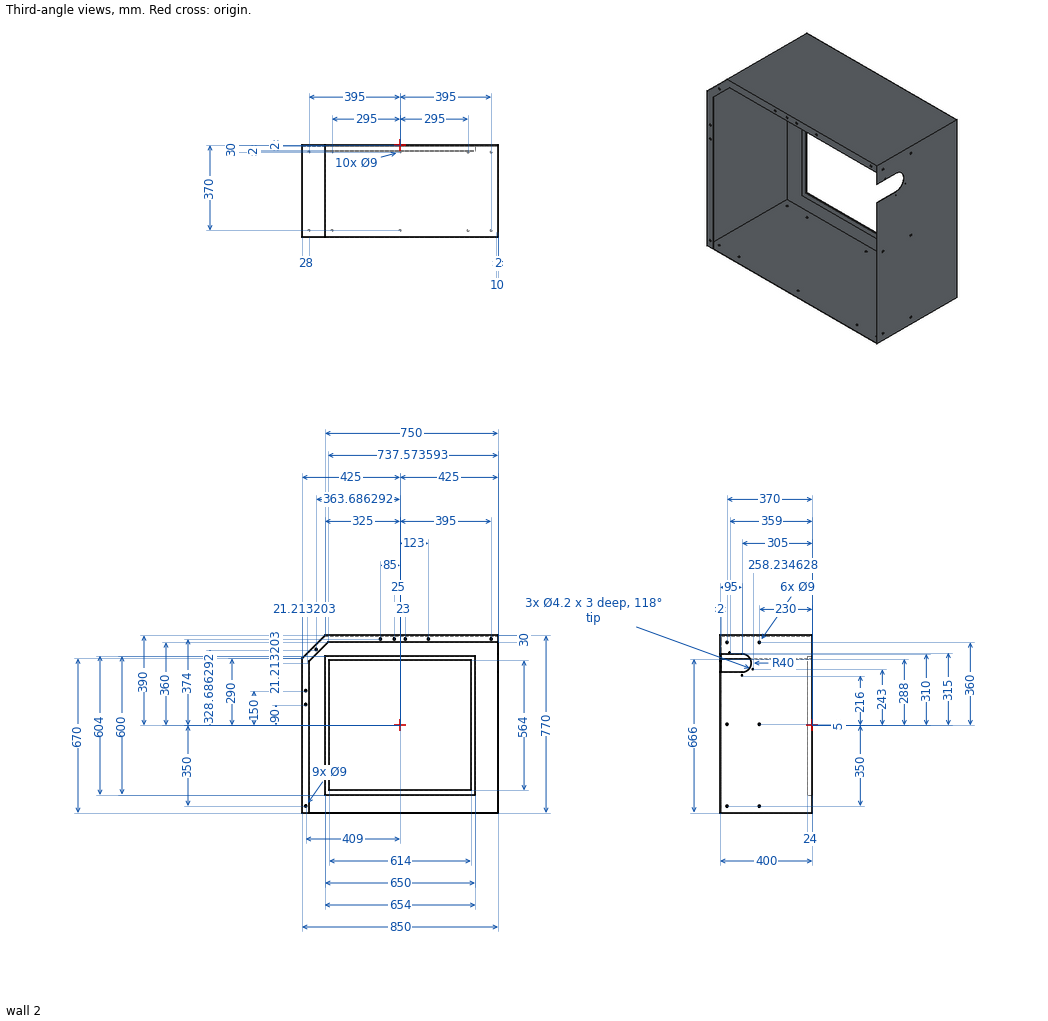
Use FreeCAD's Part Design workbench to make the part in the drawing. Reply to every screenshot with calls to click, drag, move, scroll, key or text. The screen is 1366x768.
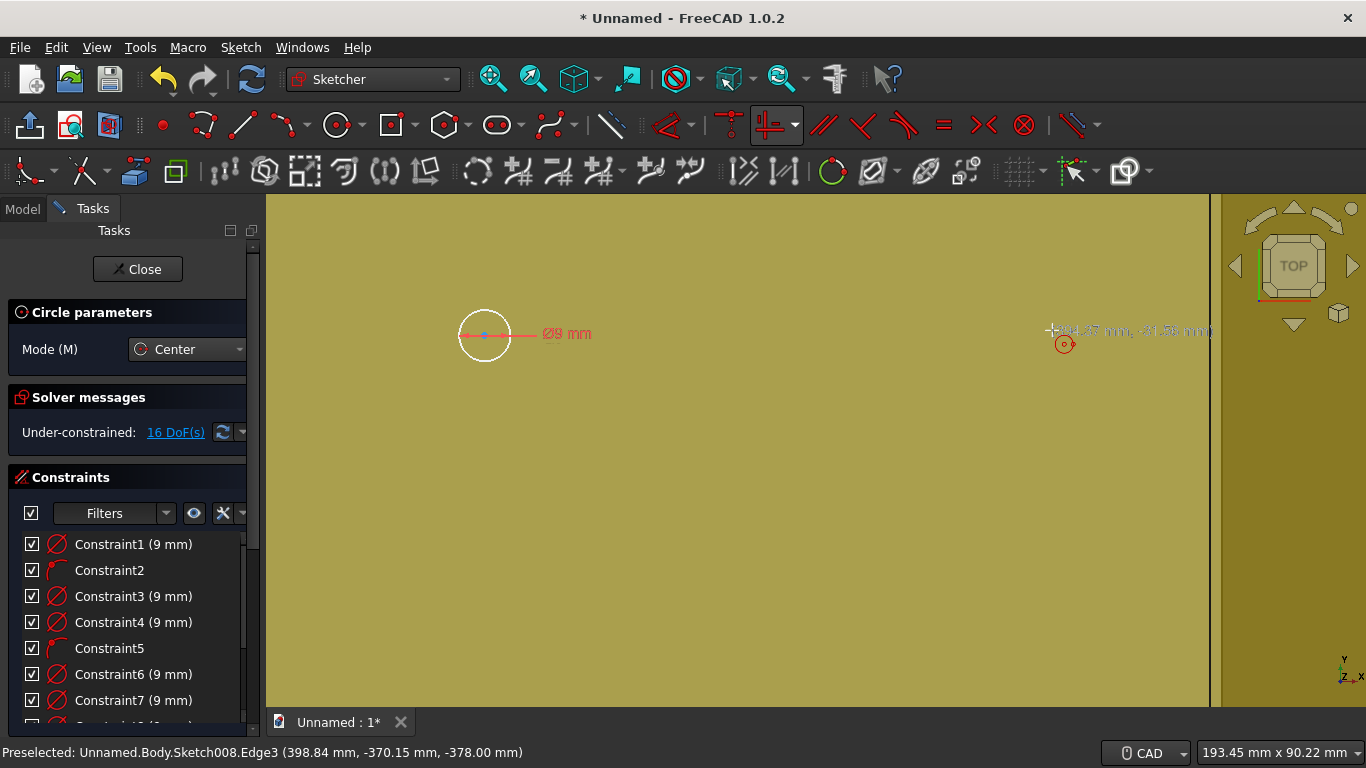
scroll(1052, 330, down, 10)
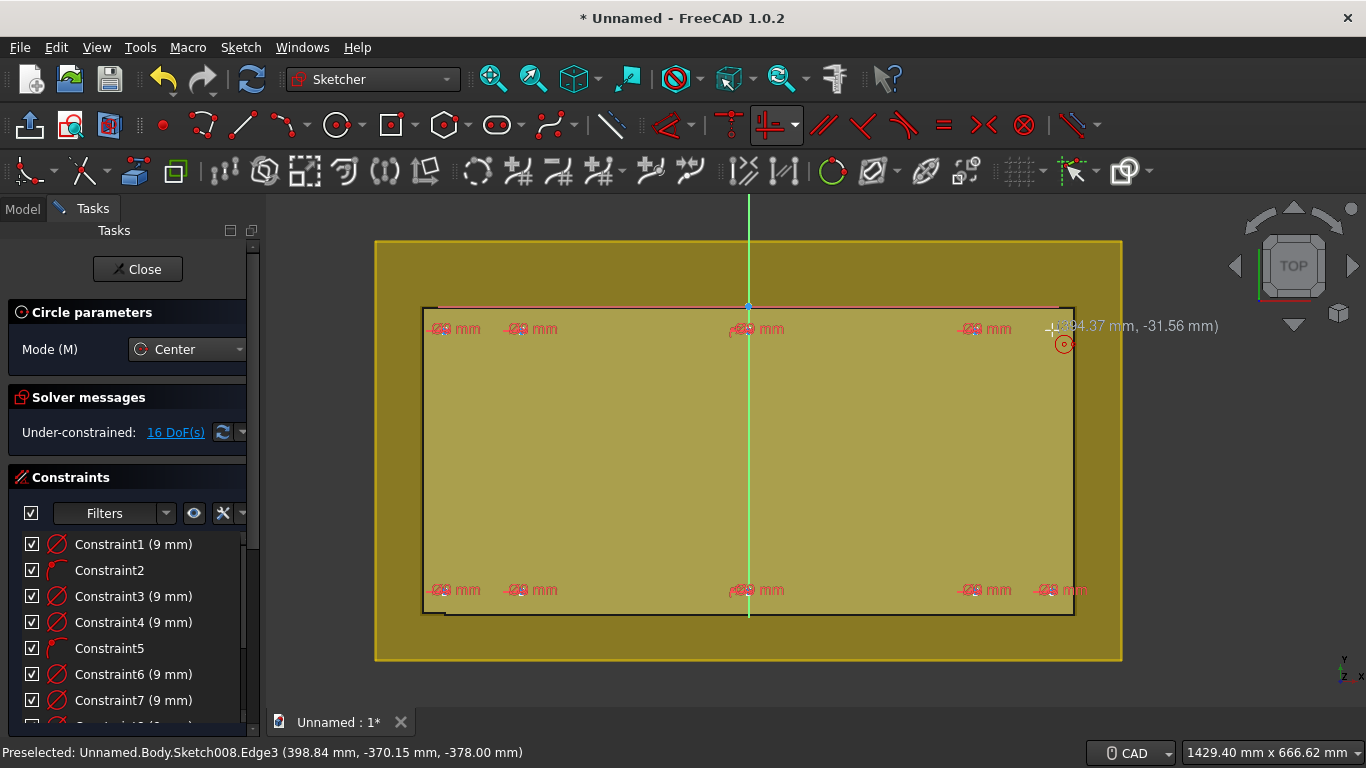
click(1052, 330)
move(1055, 327)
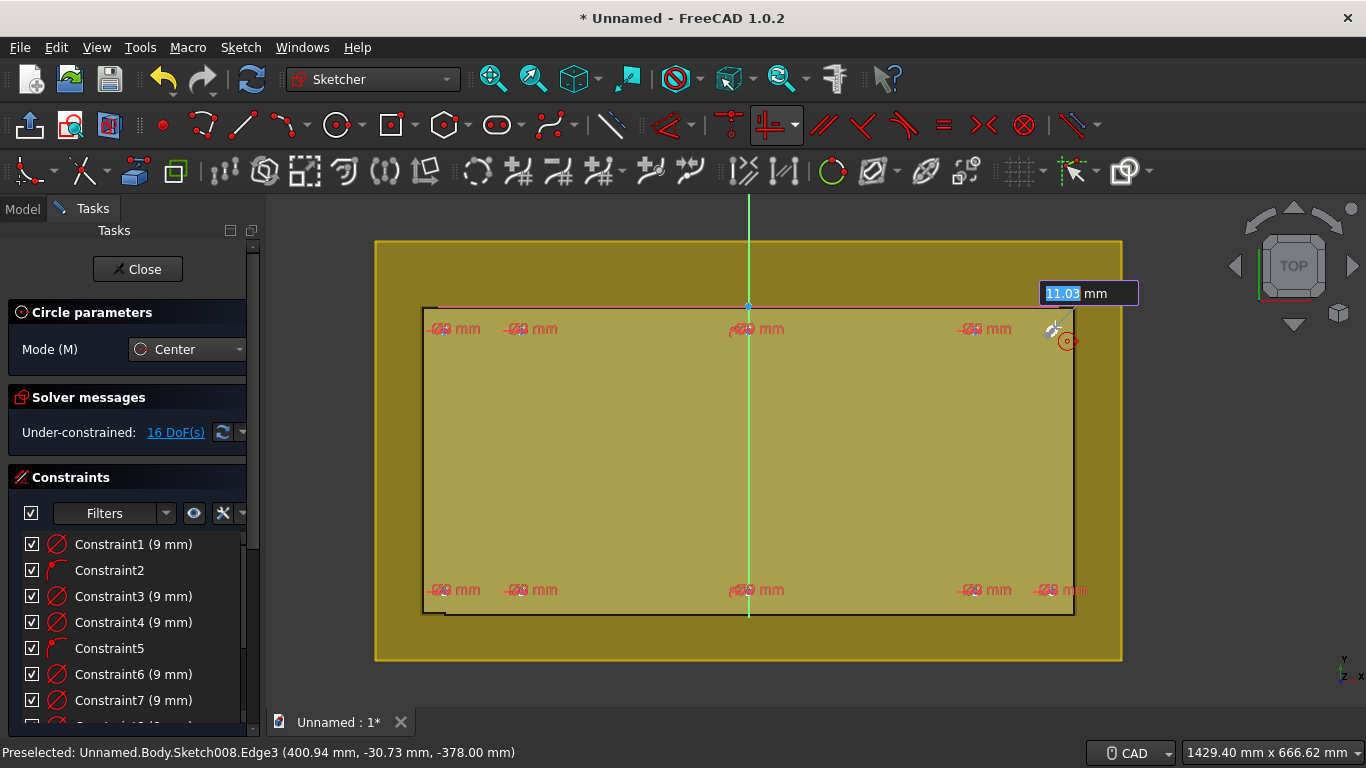
text(9)
key(Return)
key(Escape)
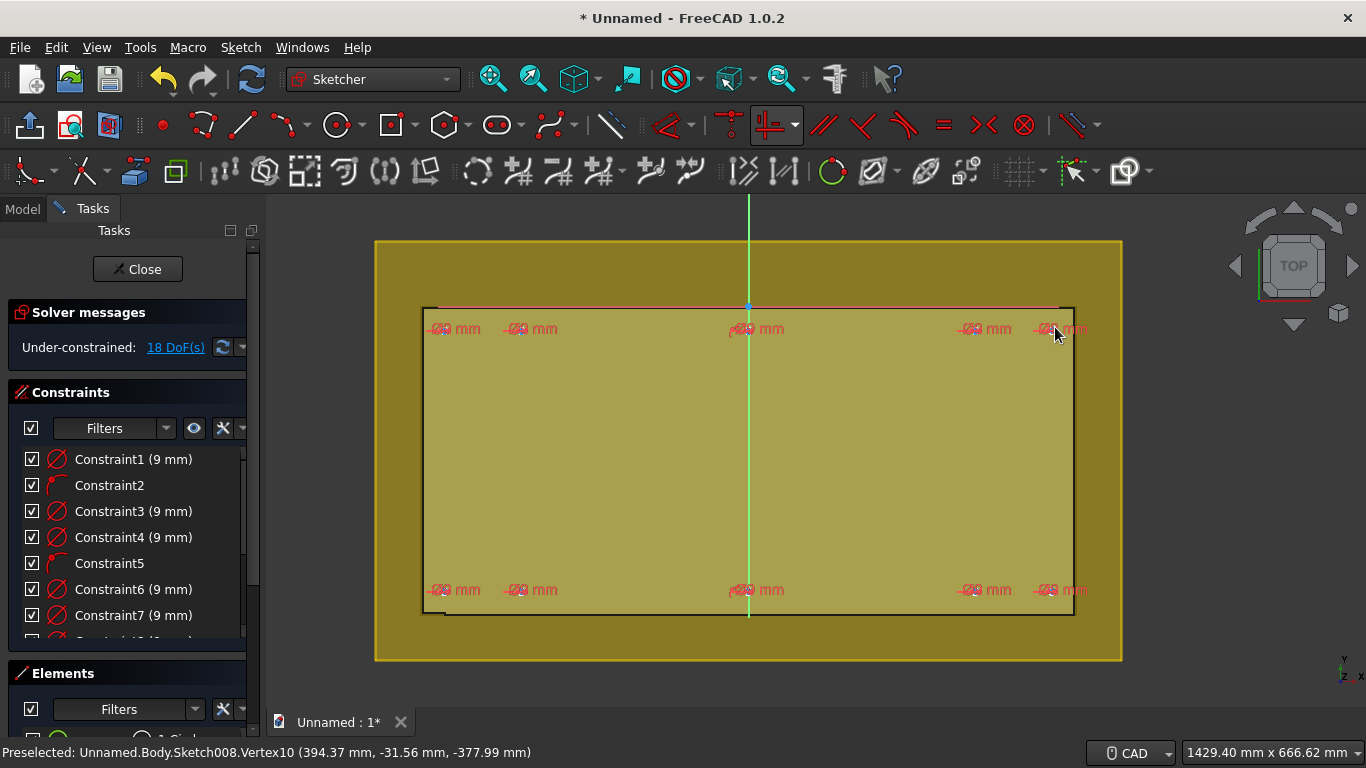
click(749, 331)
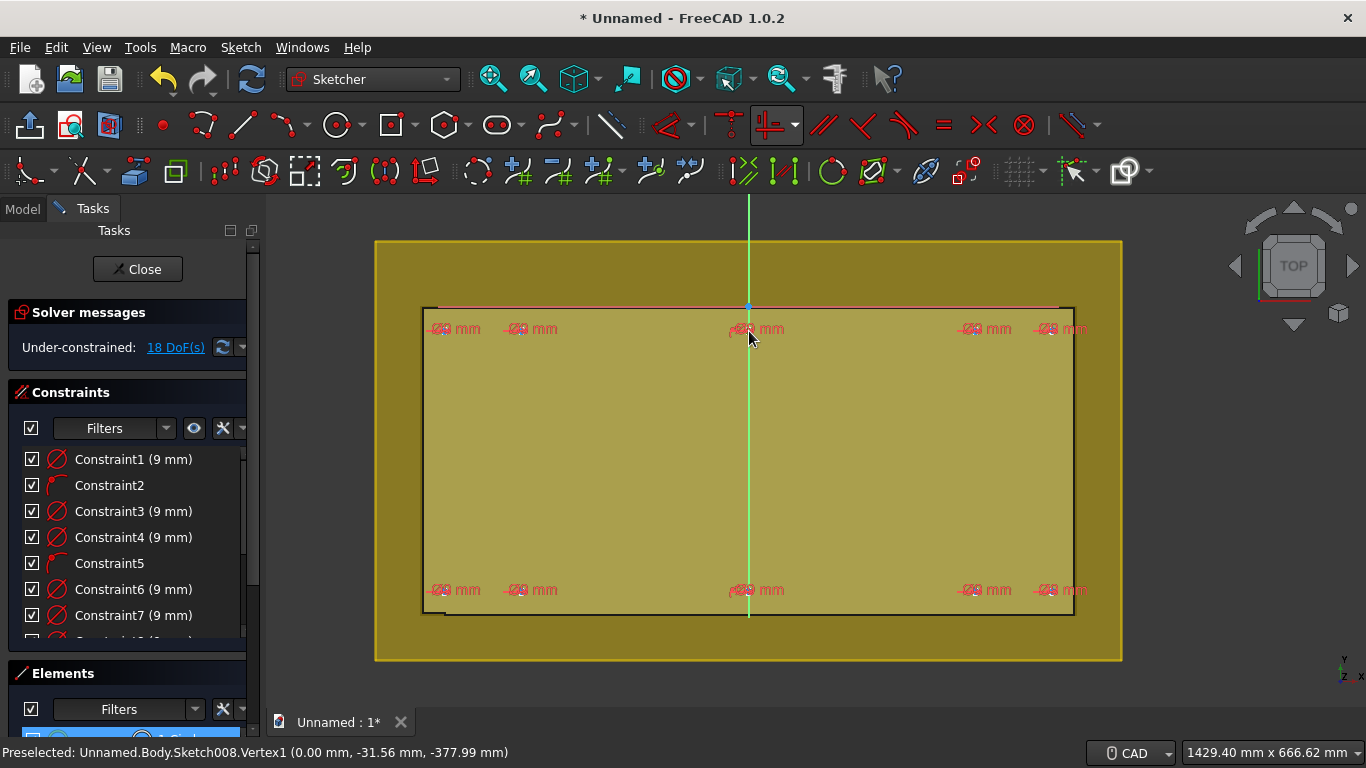
click(522, 331)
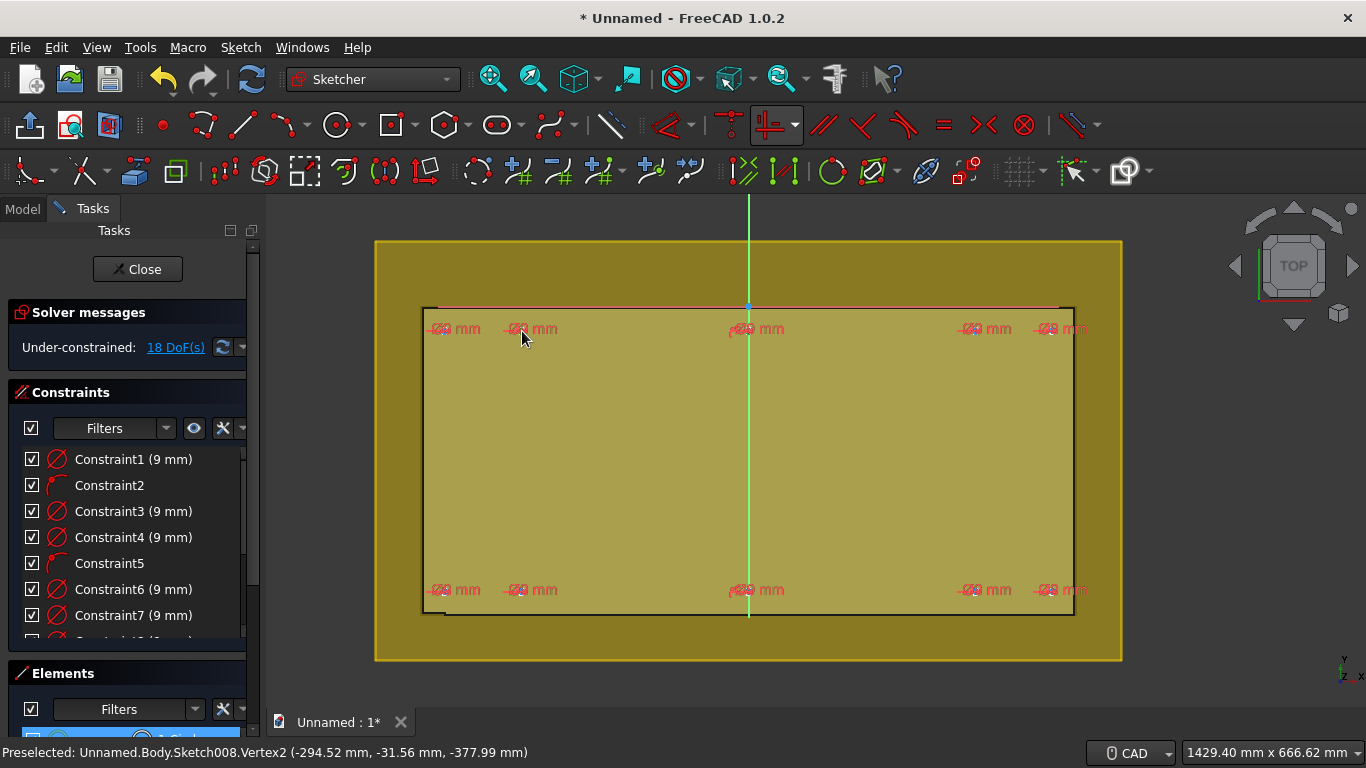
key(h)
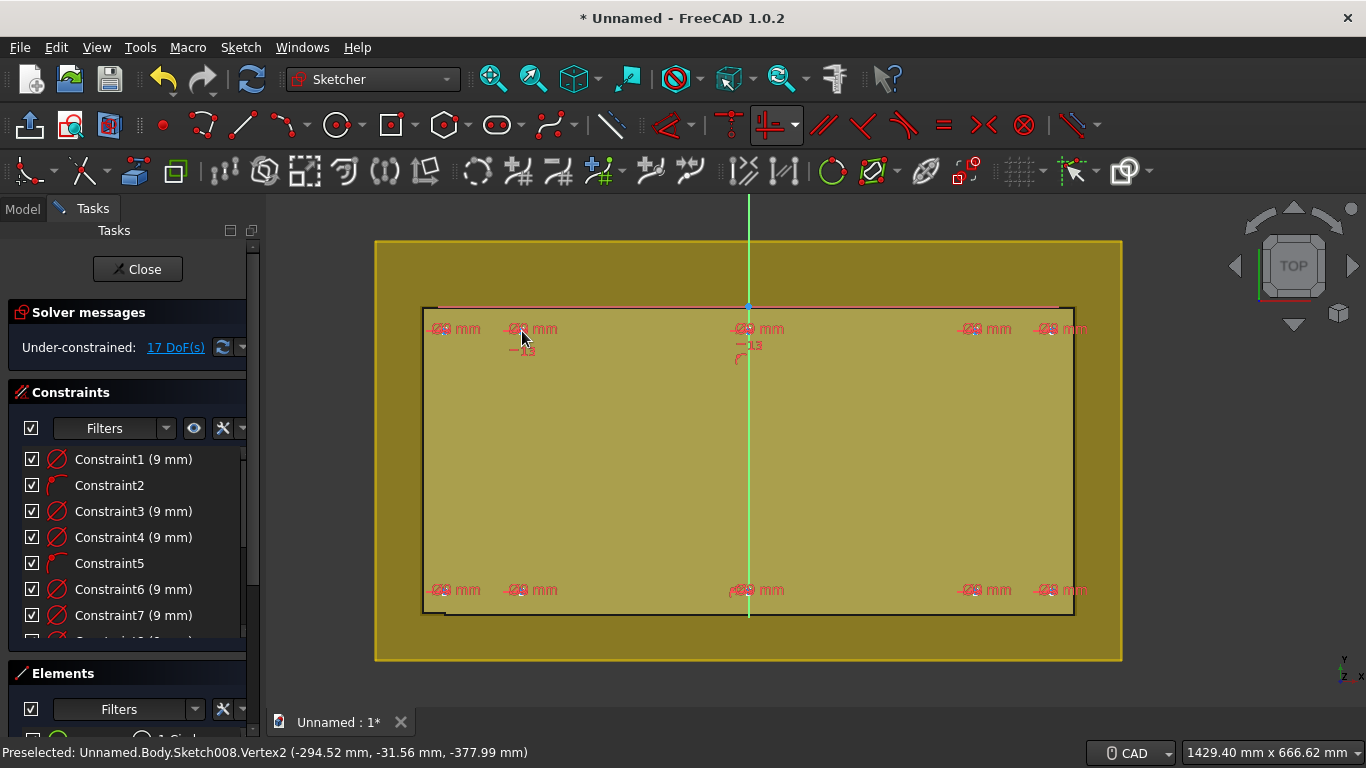
click(522, 331)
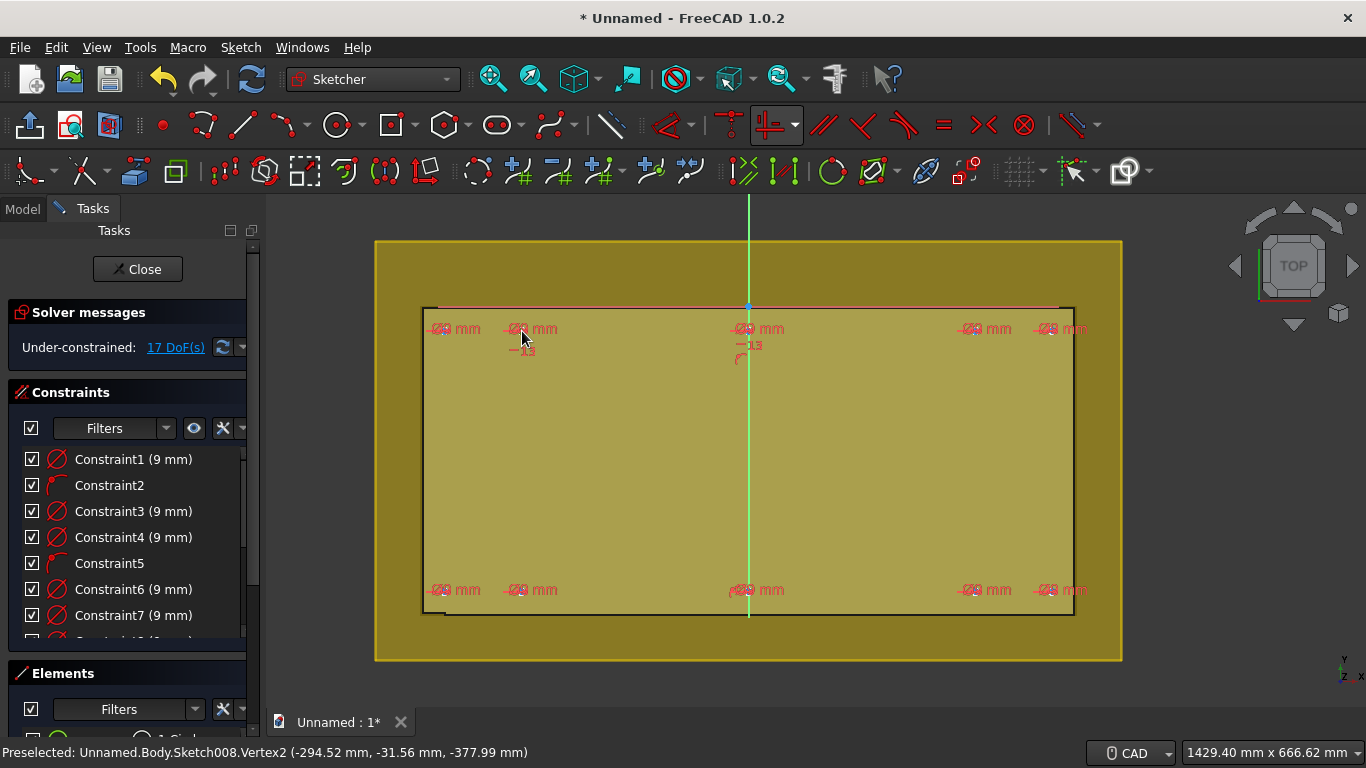
click(522, 592)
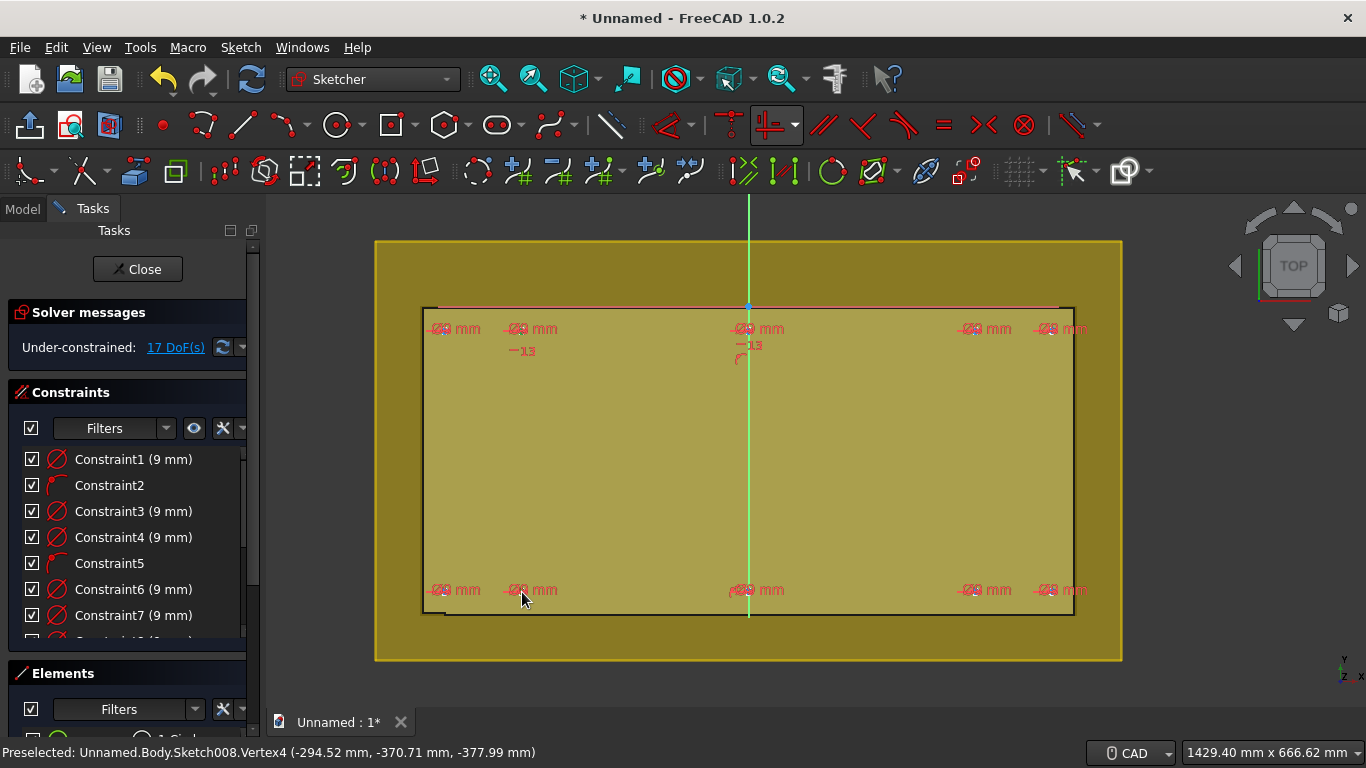
click(798, 126)